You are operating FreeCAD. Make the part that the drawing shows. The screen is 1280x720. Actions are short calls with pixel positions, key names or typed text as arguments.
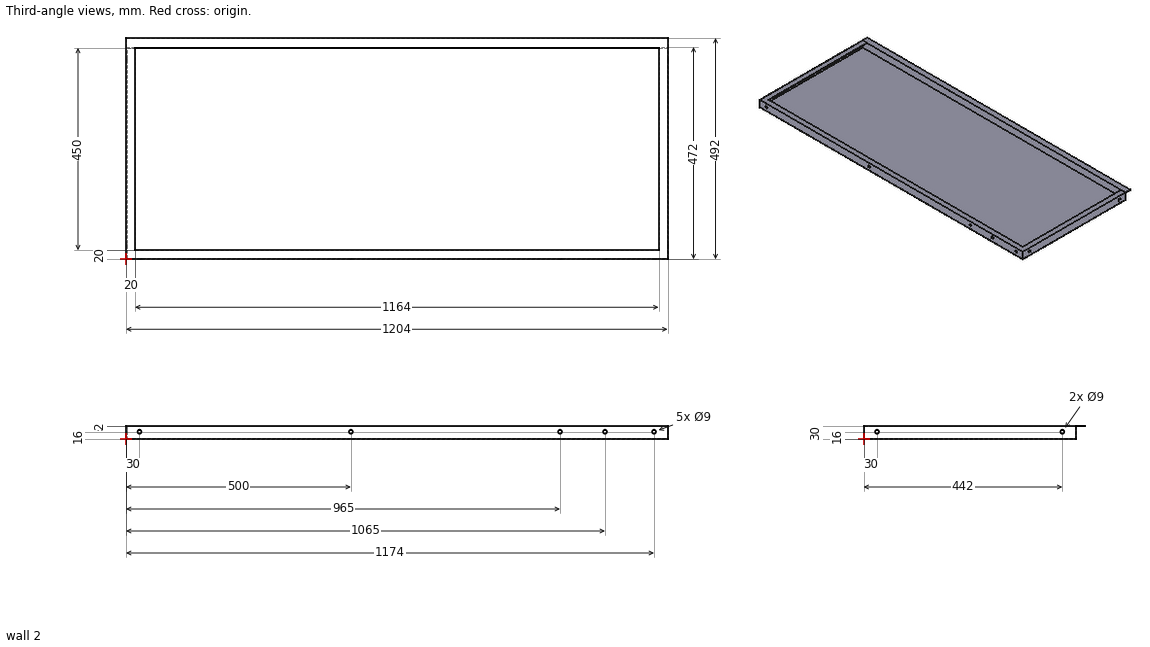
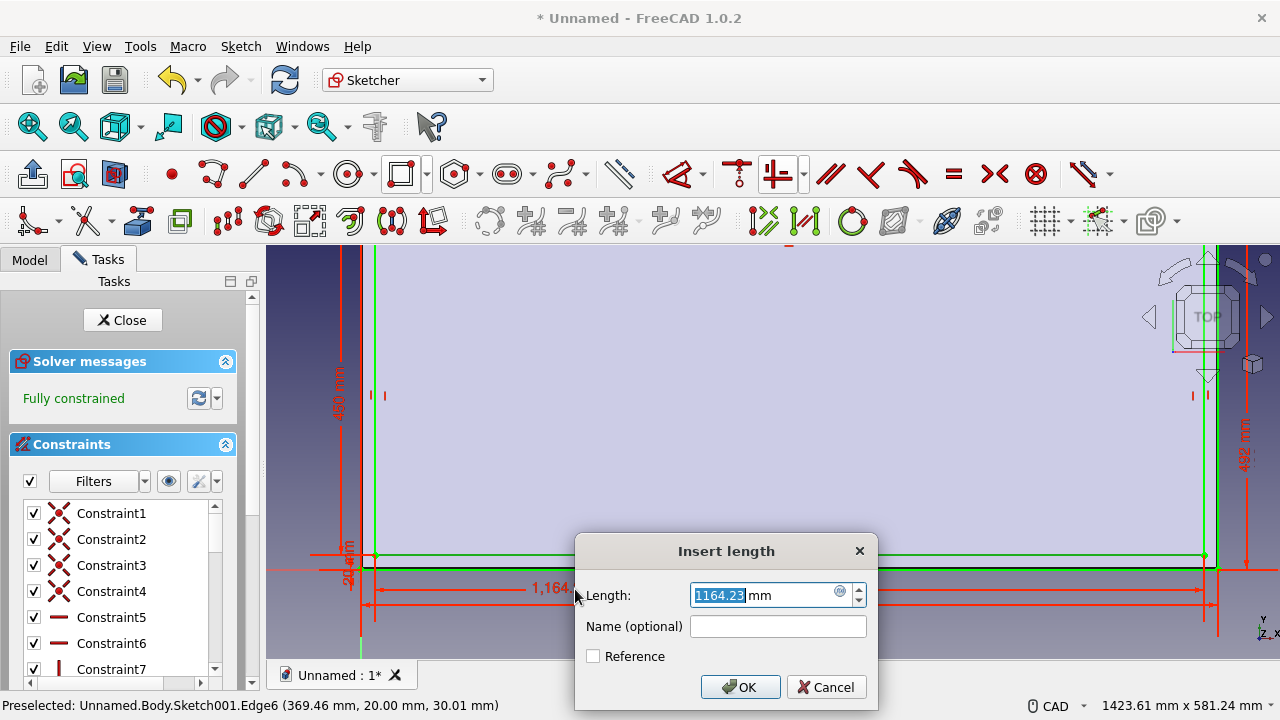
text(1164)
key(Return)
key(Escape)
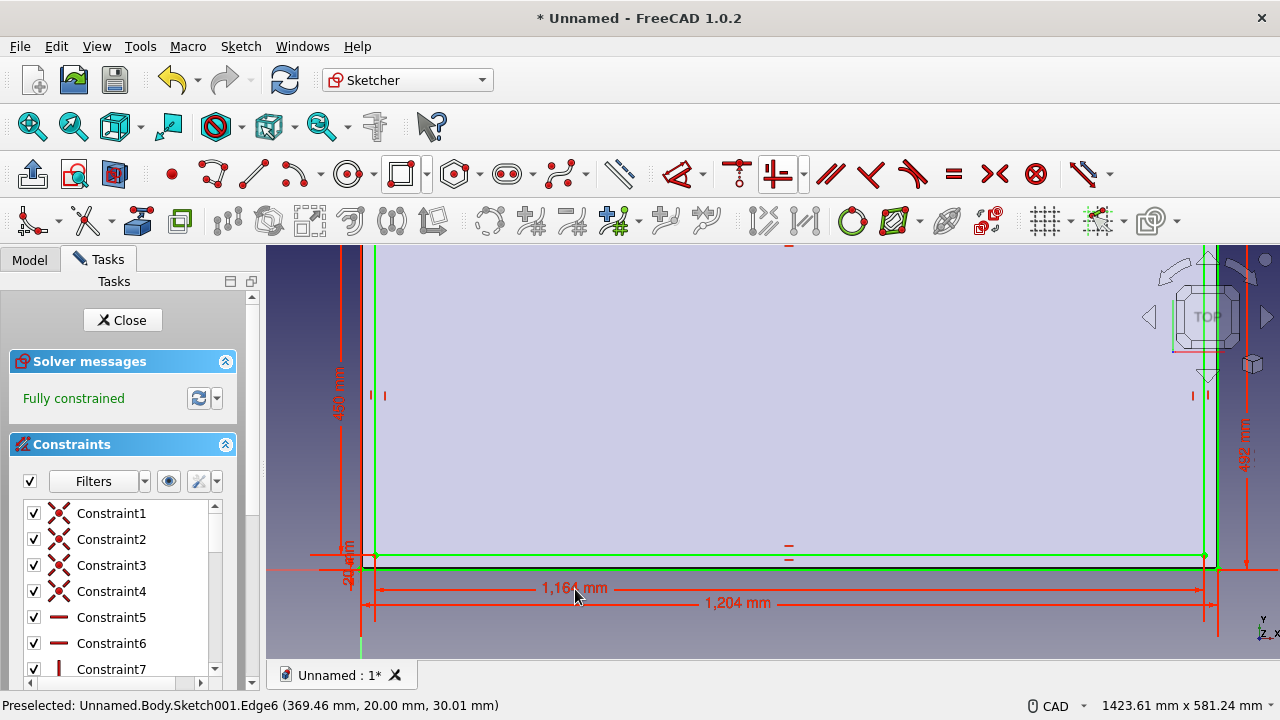
click(123, 320)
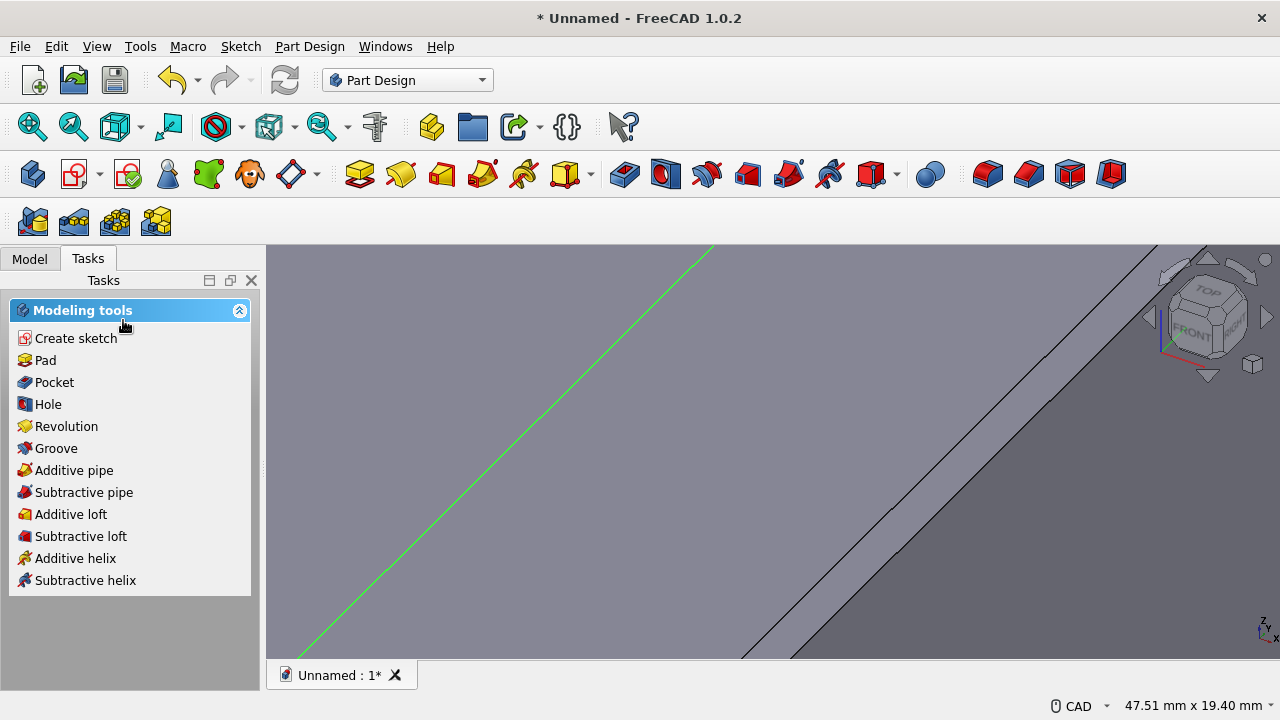
click(360, 174)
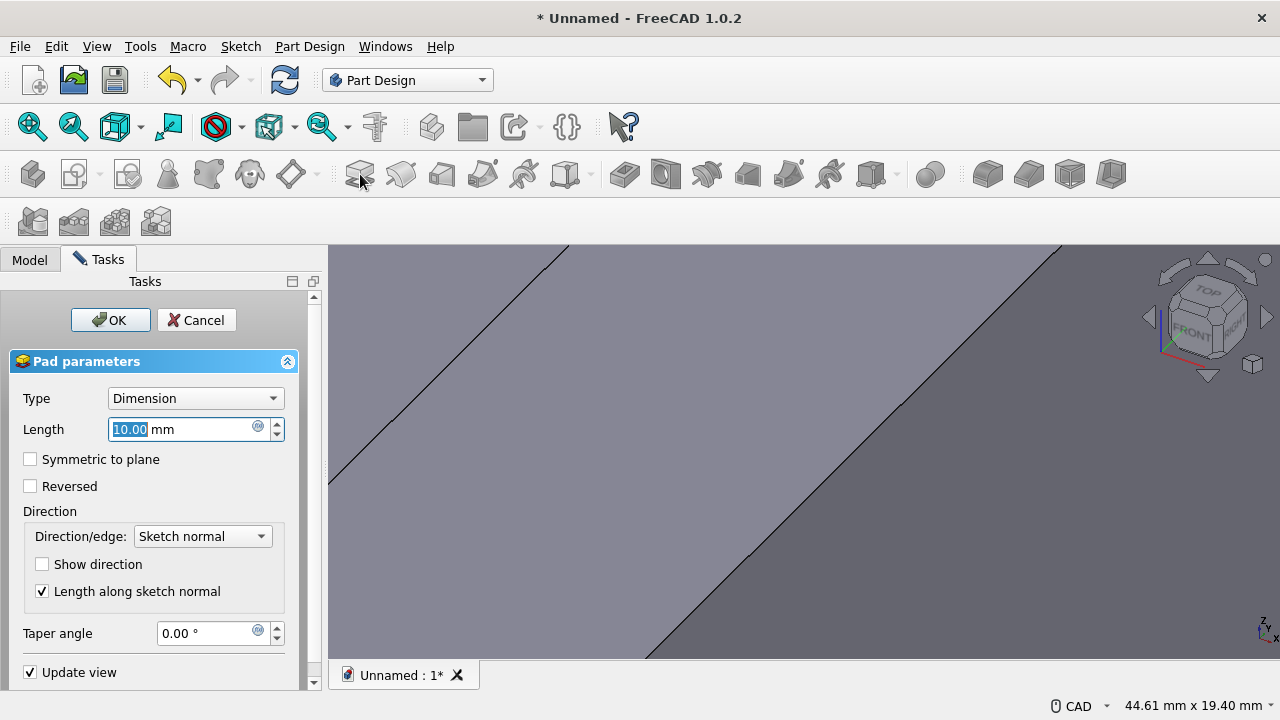
text(2)
key(Tab)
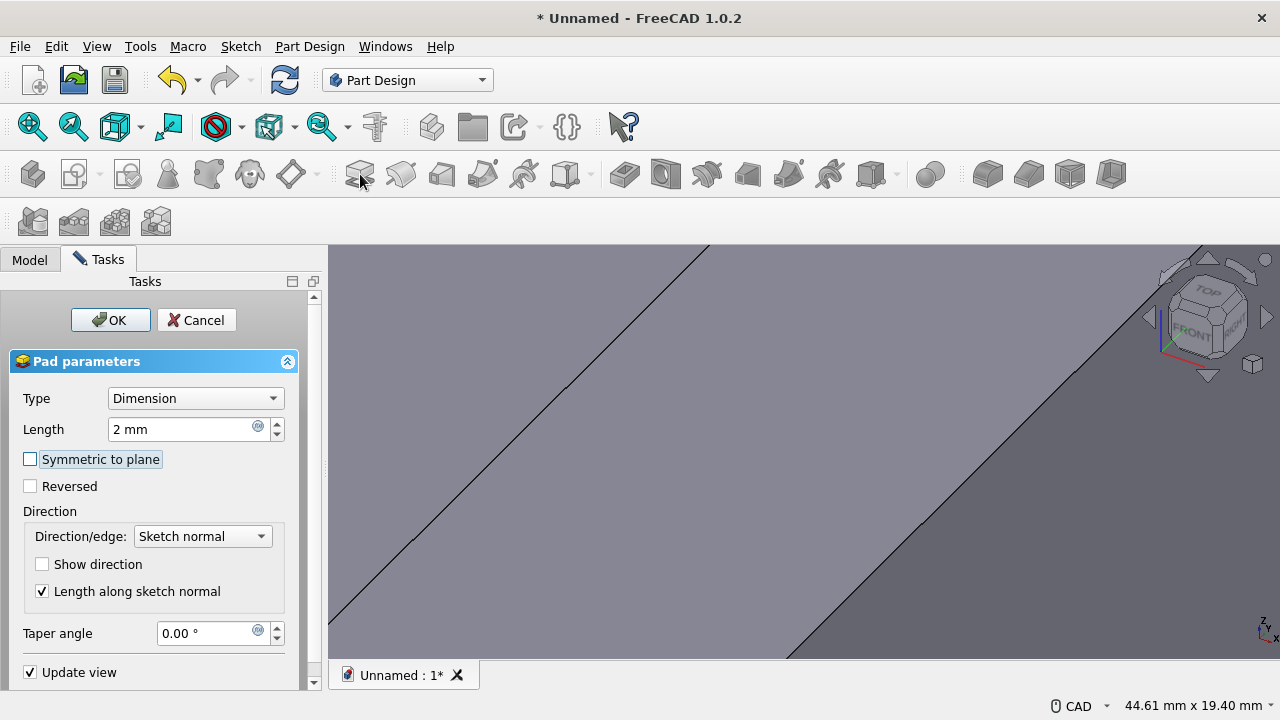
click(31, 486)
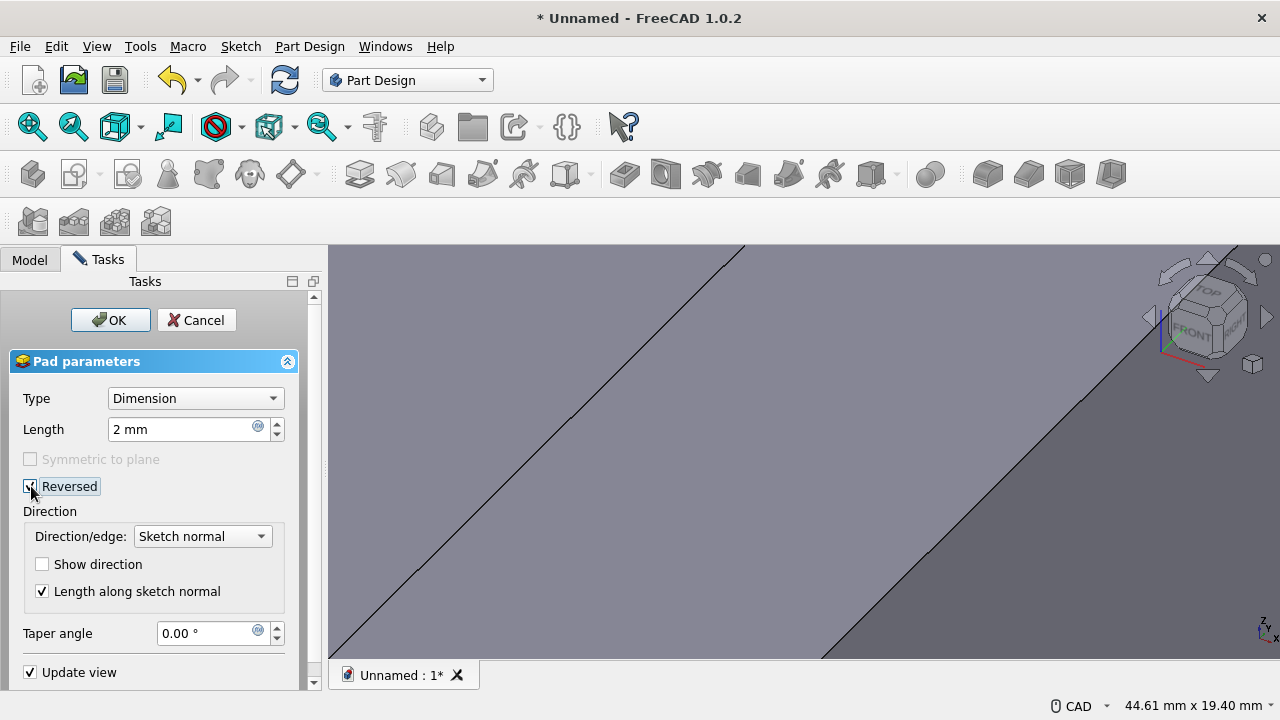
click(111, 320)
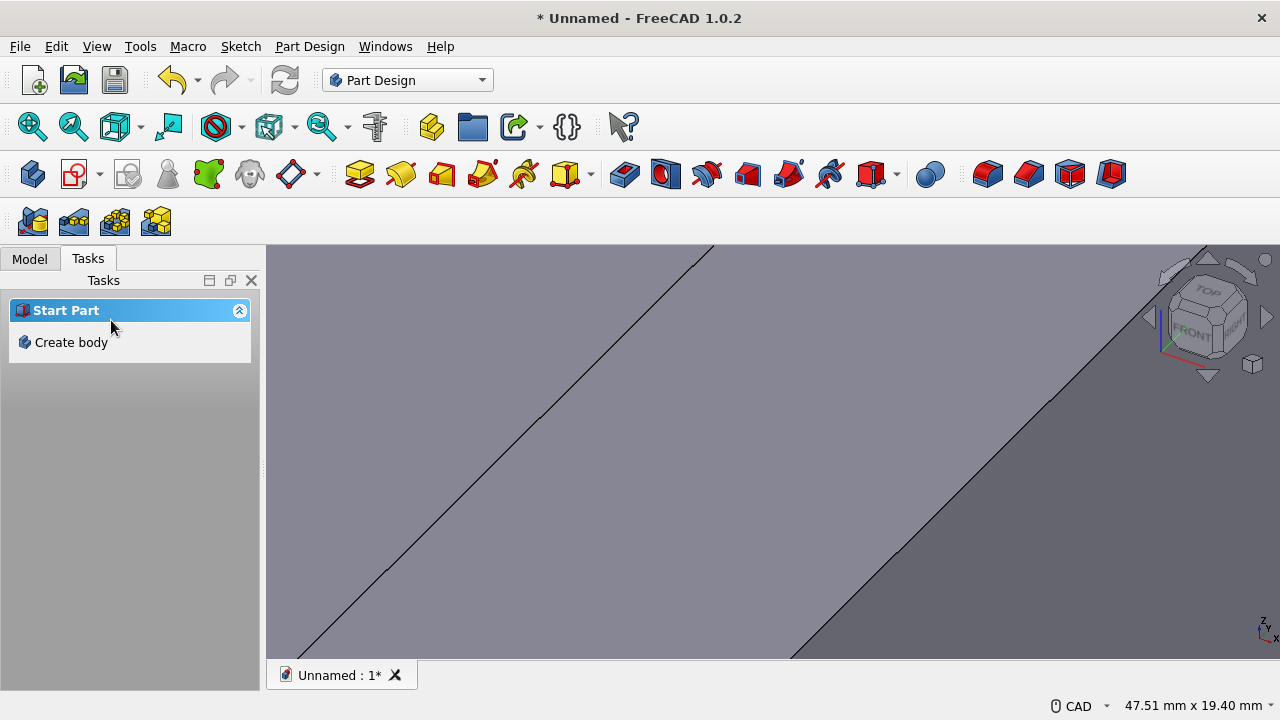
key(v)
key(f)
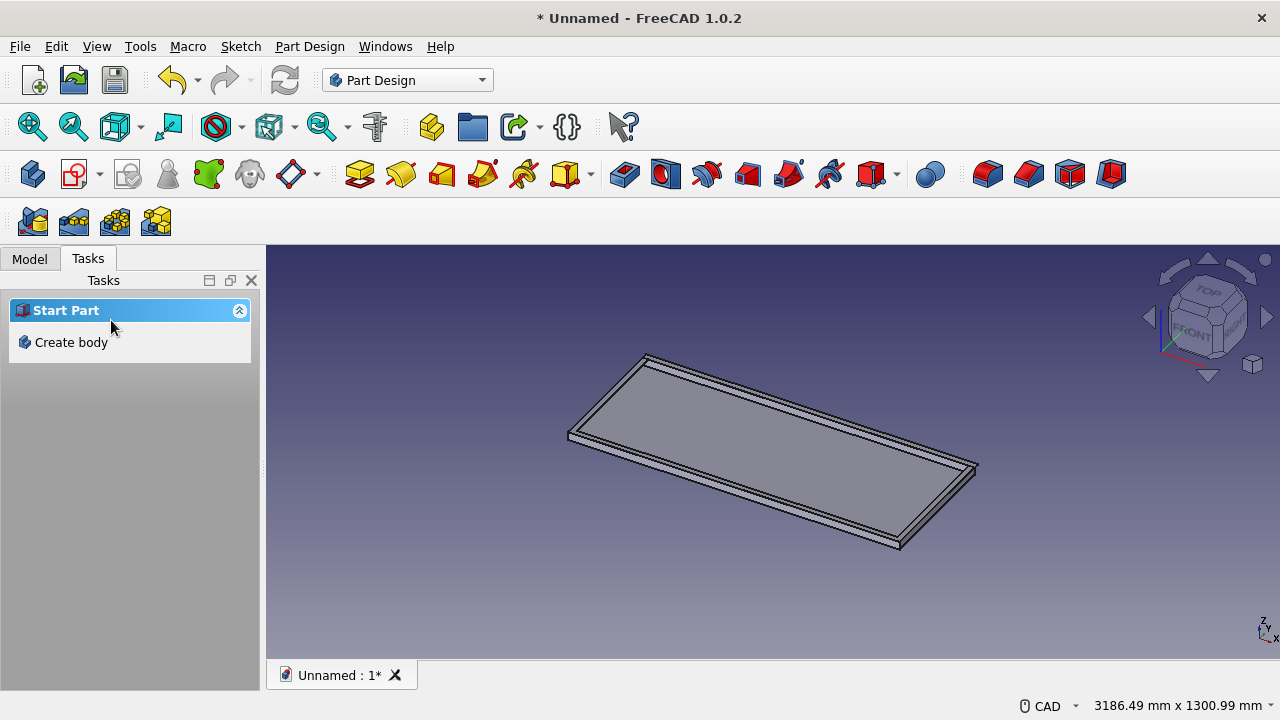
click(30, 258)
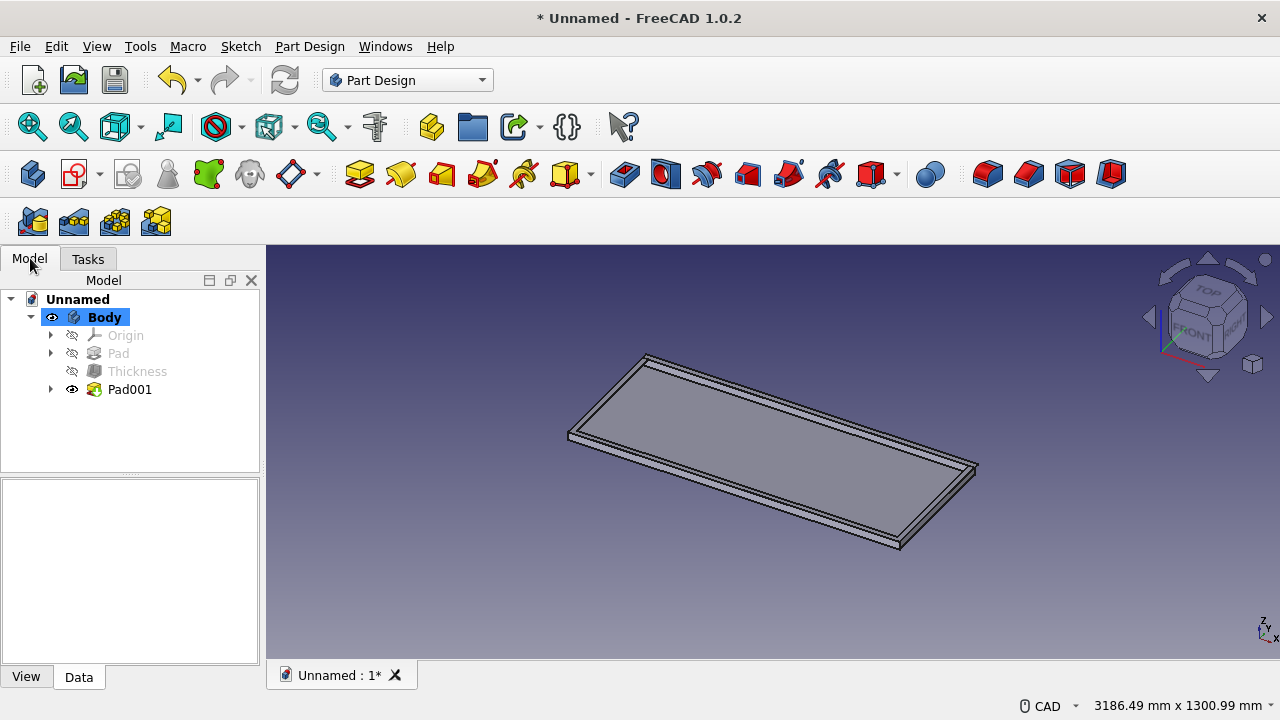
click(51, 335)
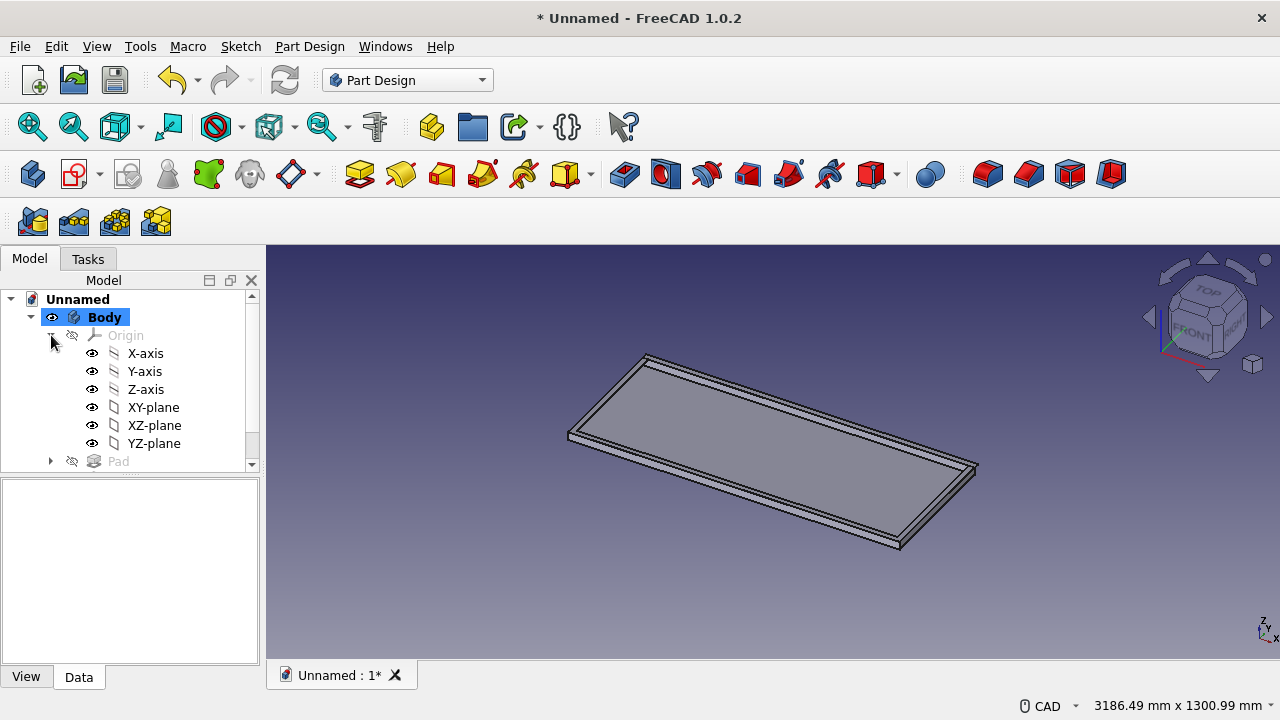
click(137, 443)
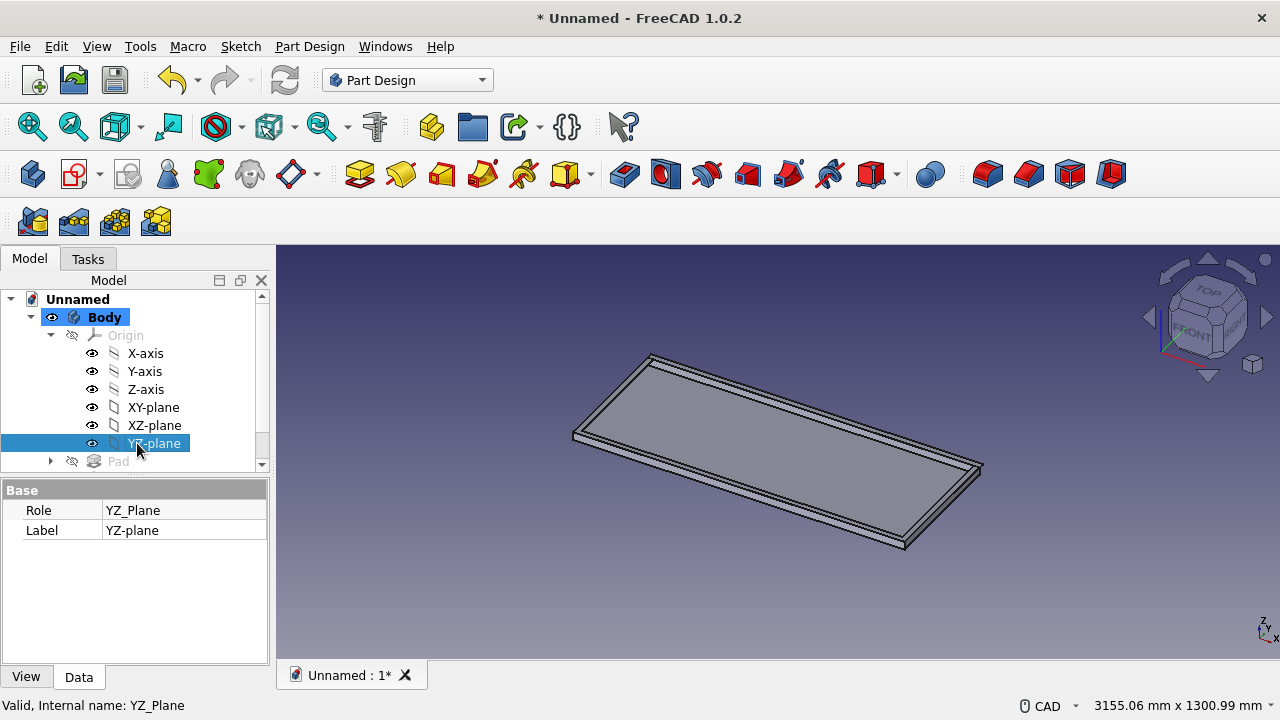
click(290, 174)